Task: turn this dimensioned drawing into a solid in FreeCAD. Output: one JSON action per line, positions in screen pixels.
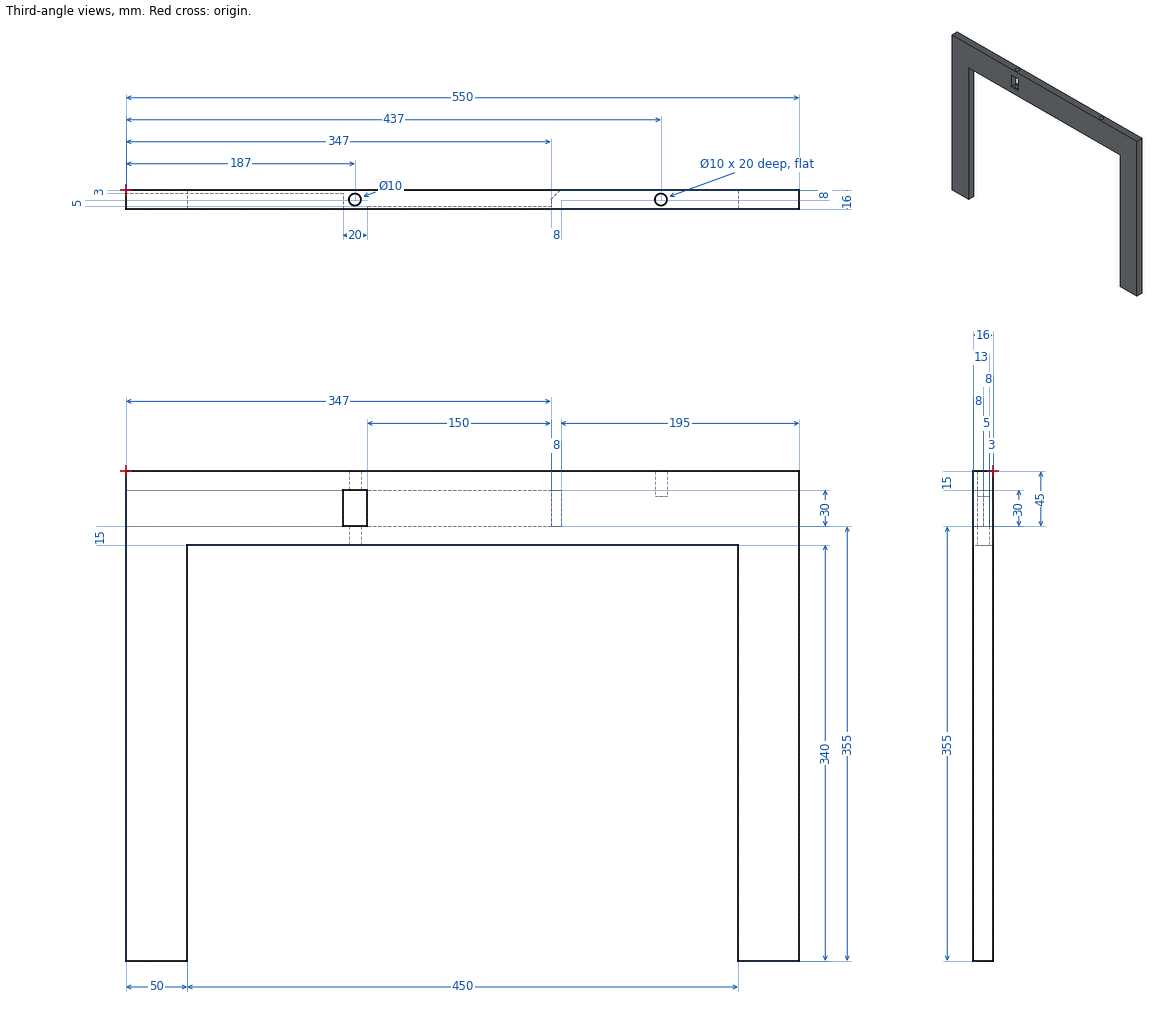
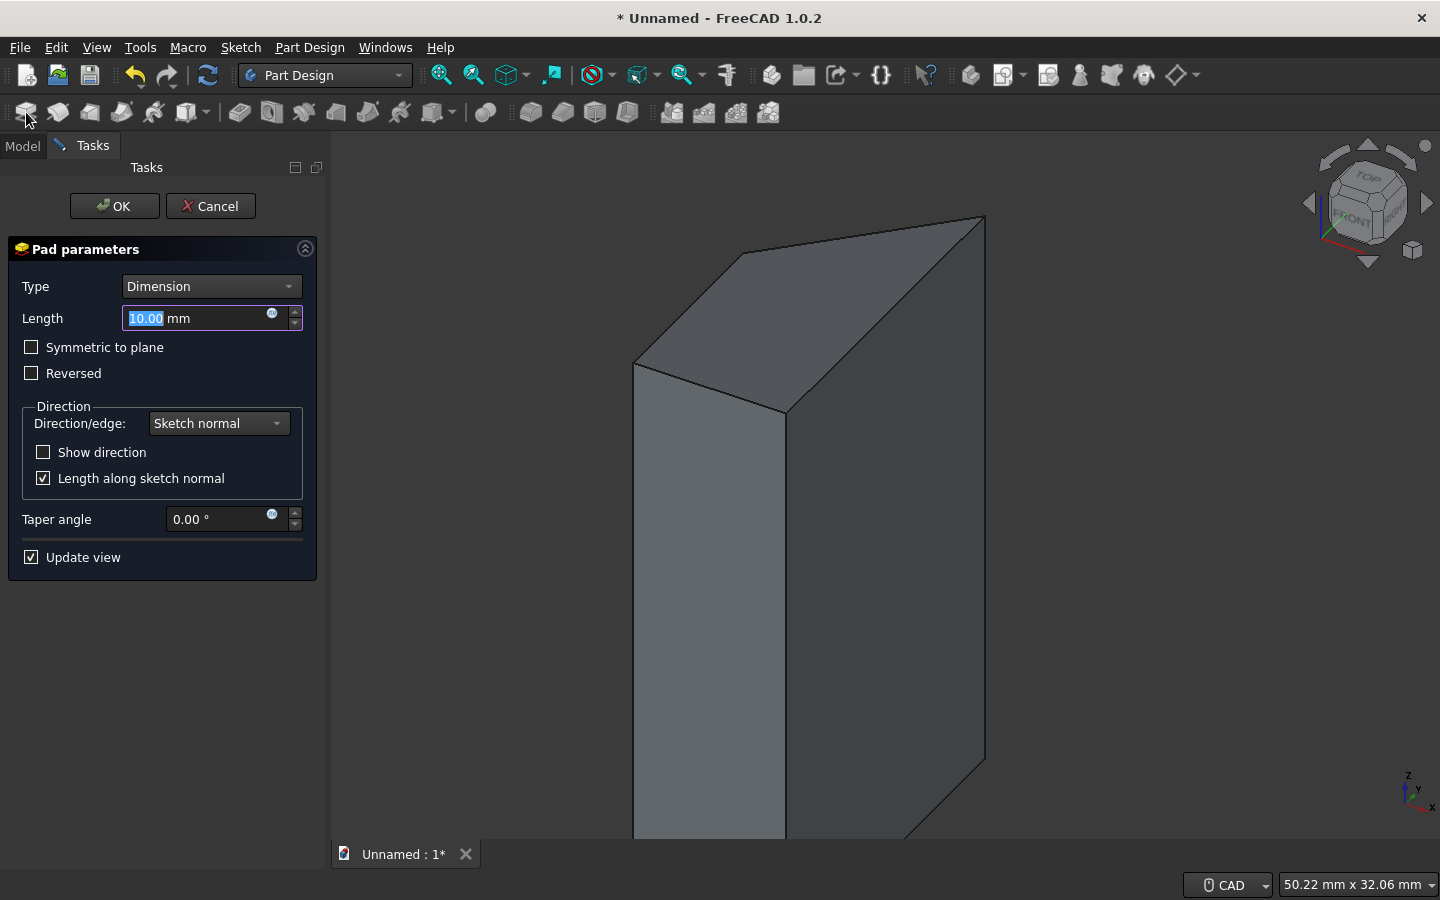
{"action": "type", "text": "8"}
{"action": "key", "text": "Tab"}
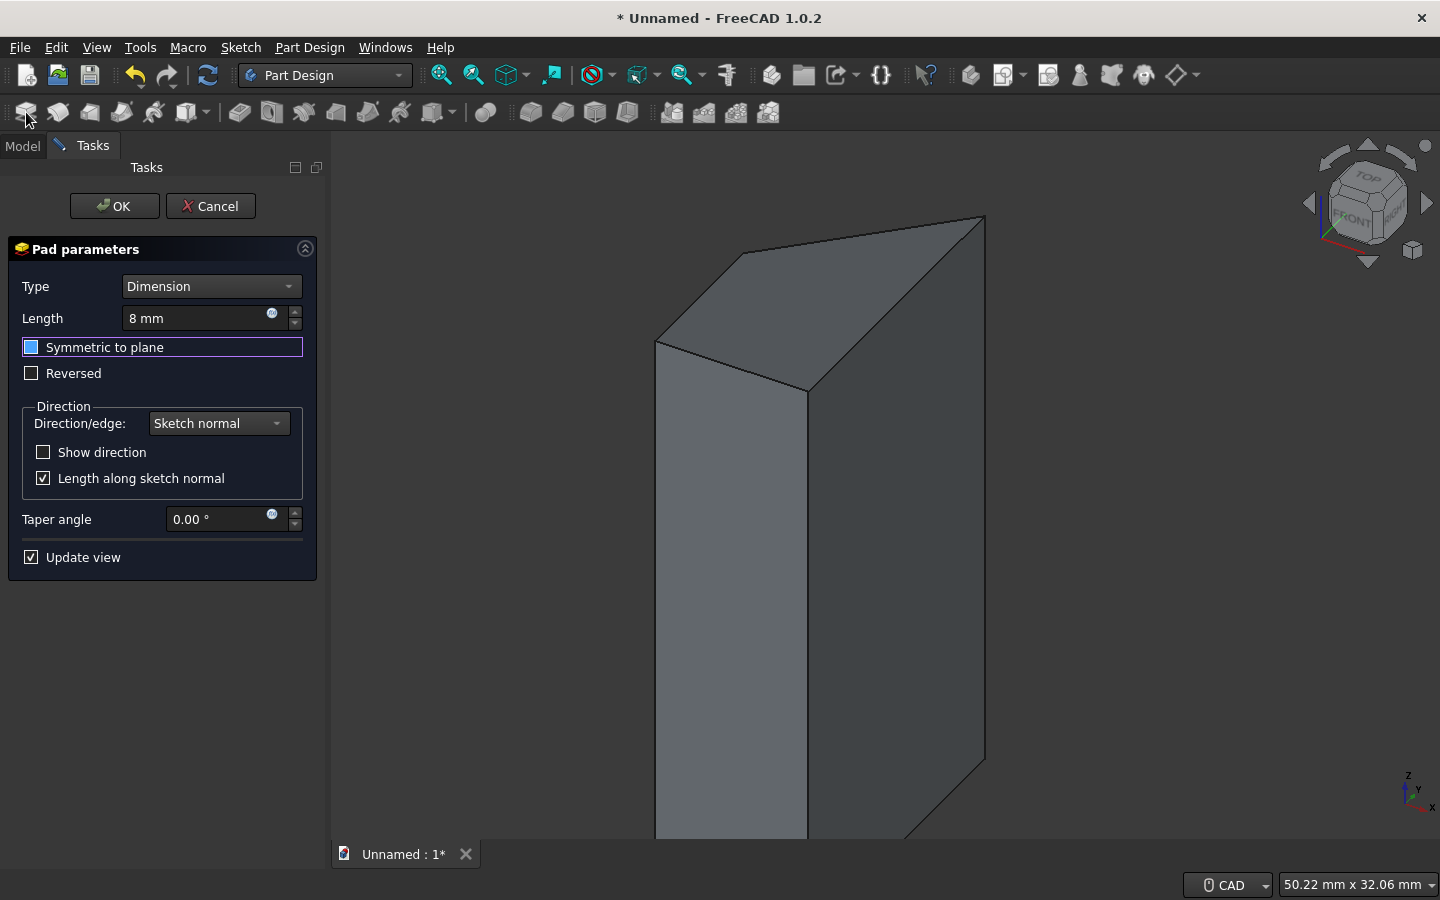
{"action": "left_click", "coordinate": [115, 206]}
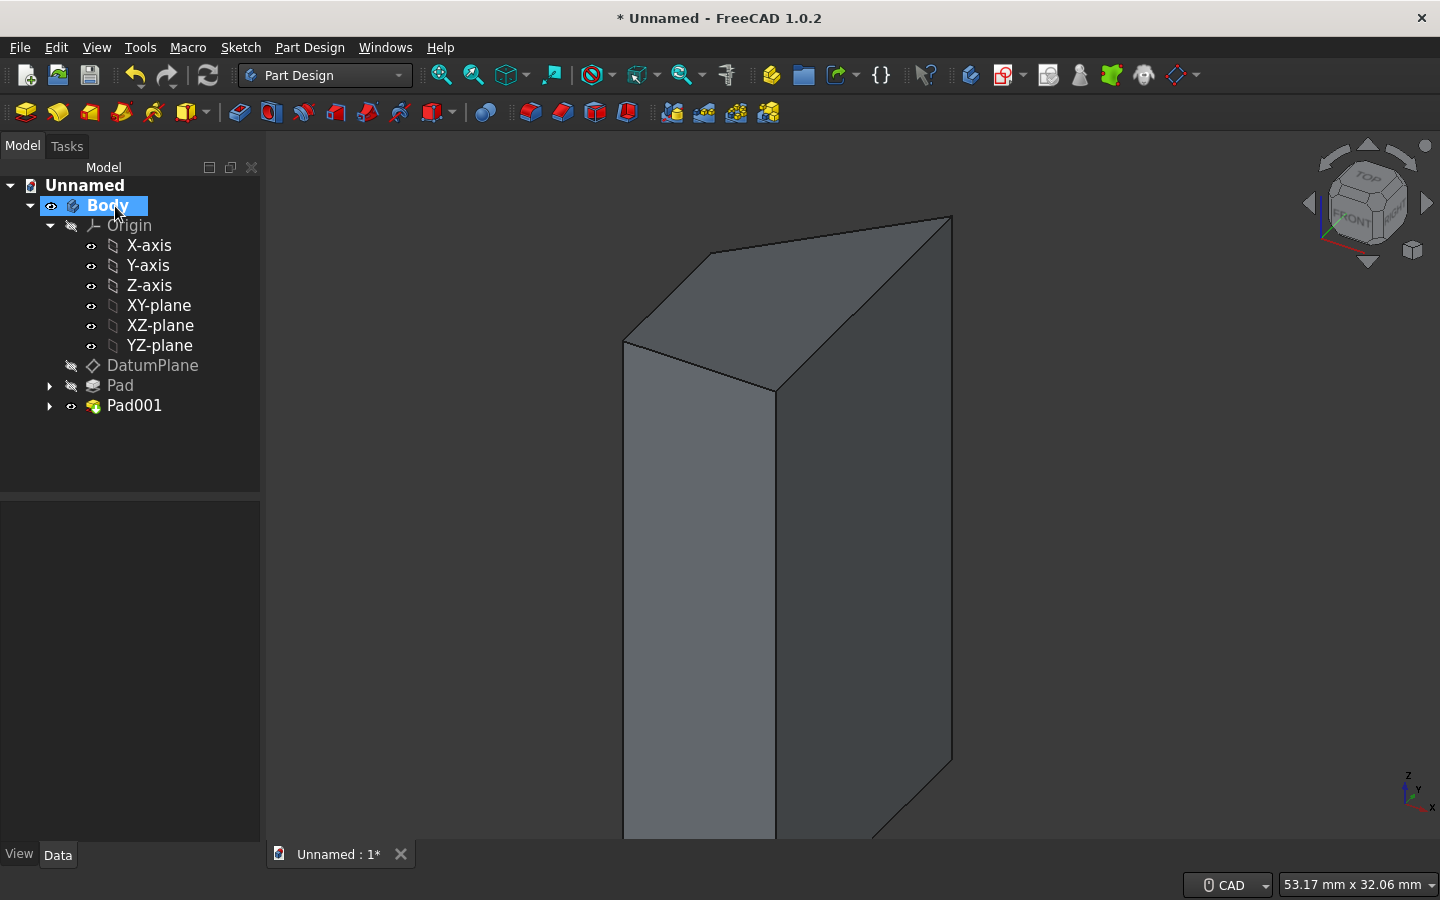
{"action": "left_click", "coordinate": [442, 76]}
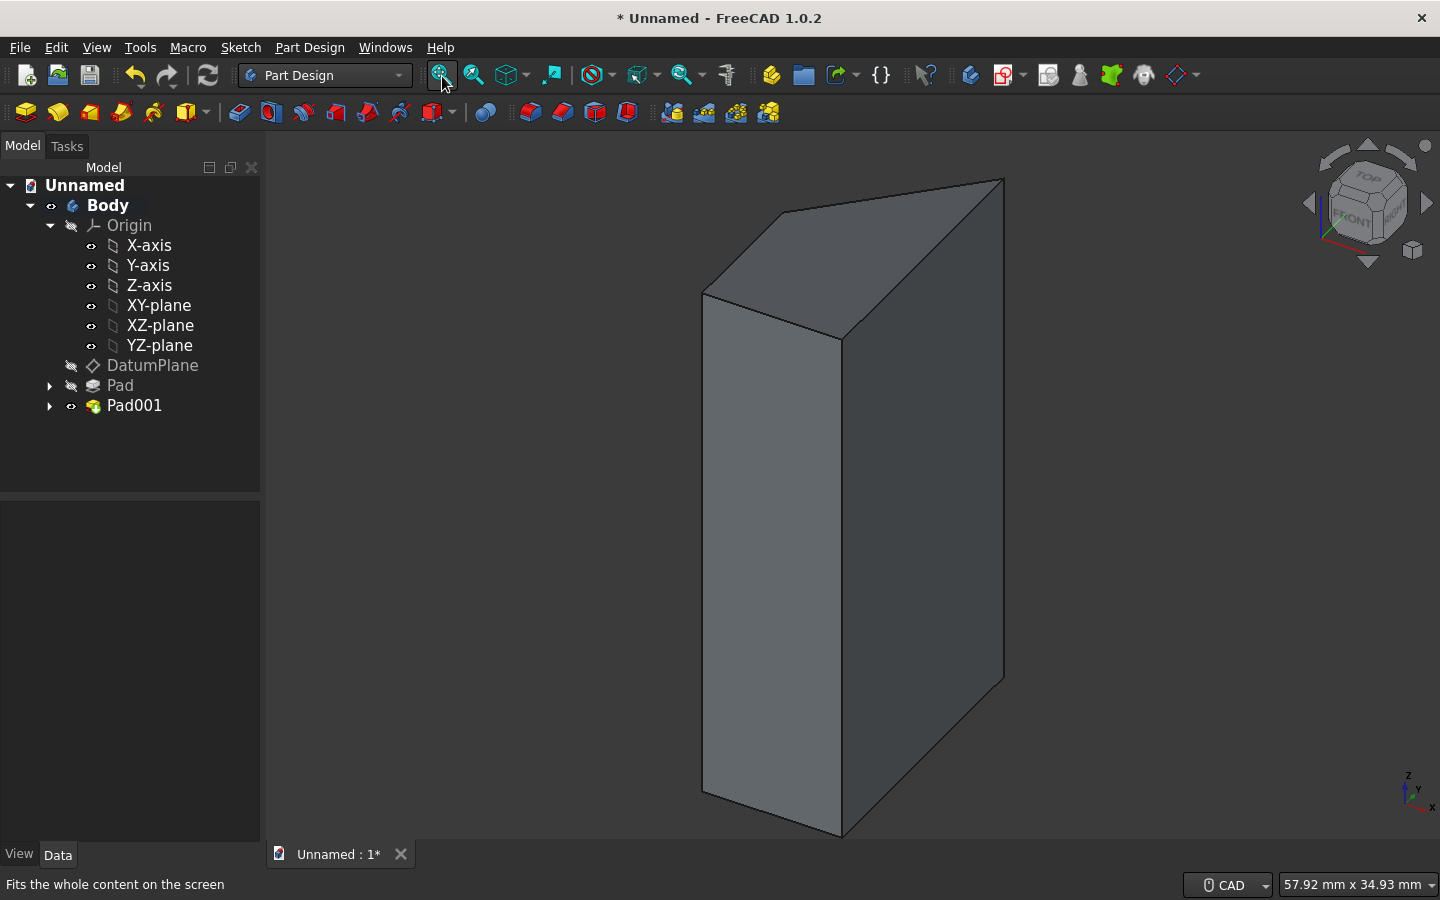
{"action": "left_click", "coordinate": [830, 258]}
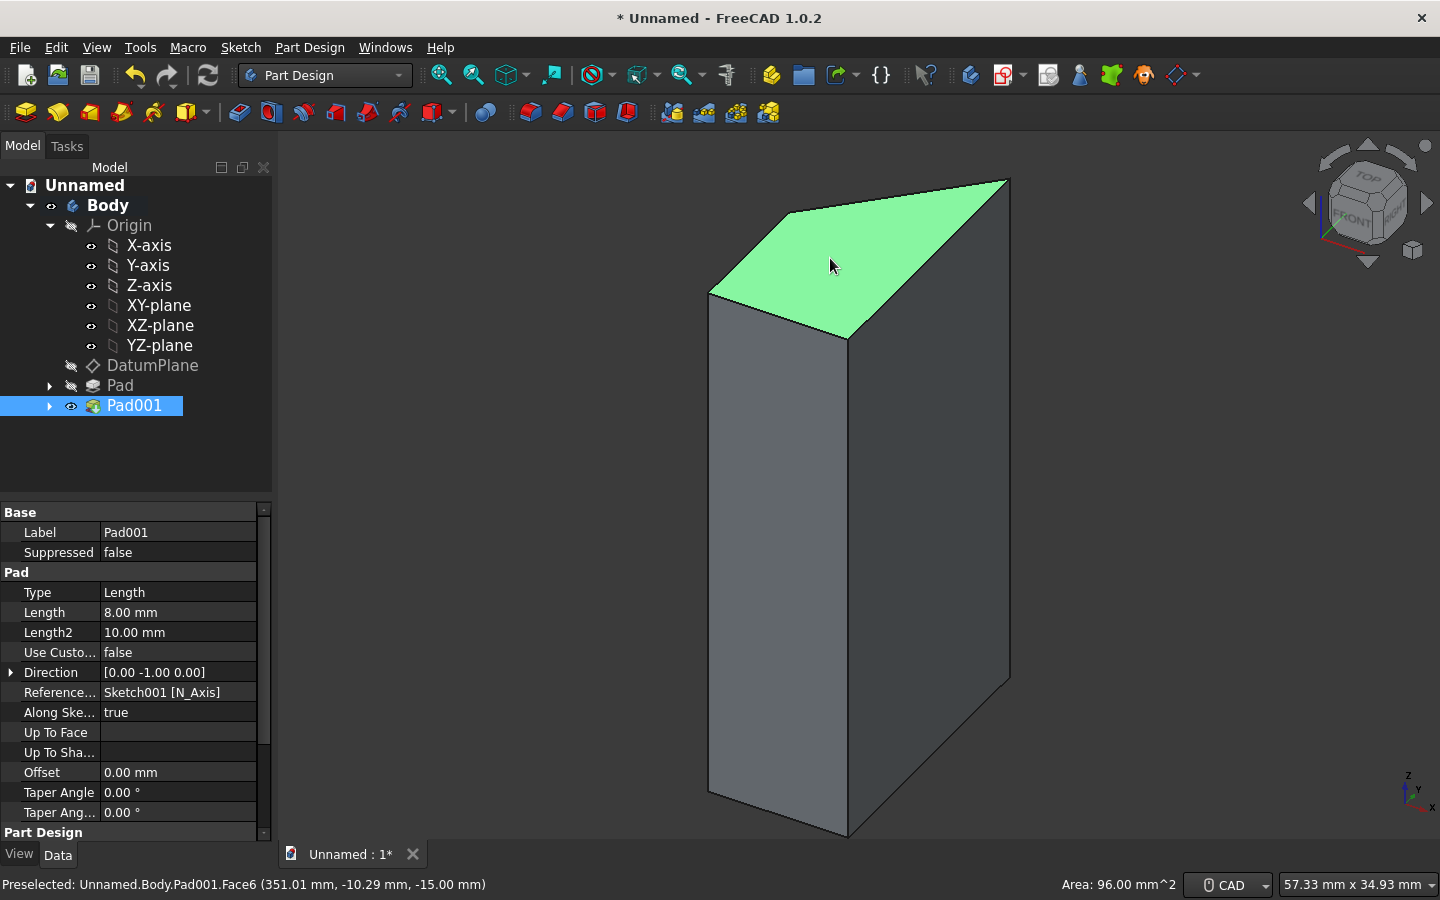
{"action": "left_click", "coordinate": [1004, 76]}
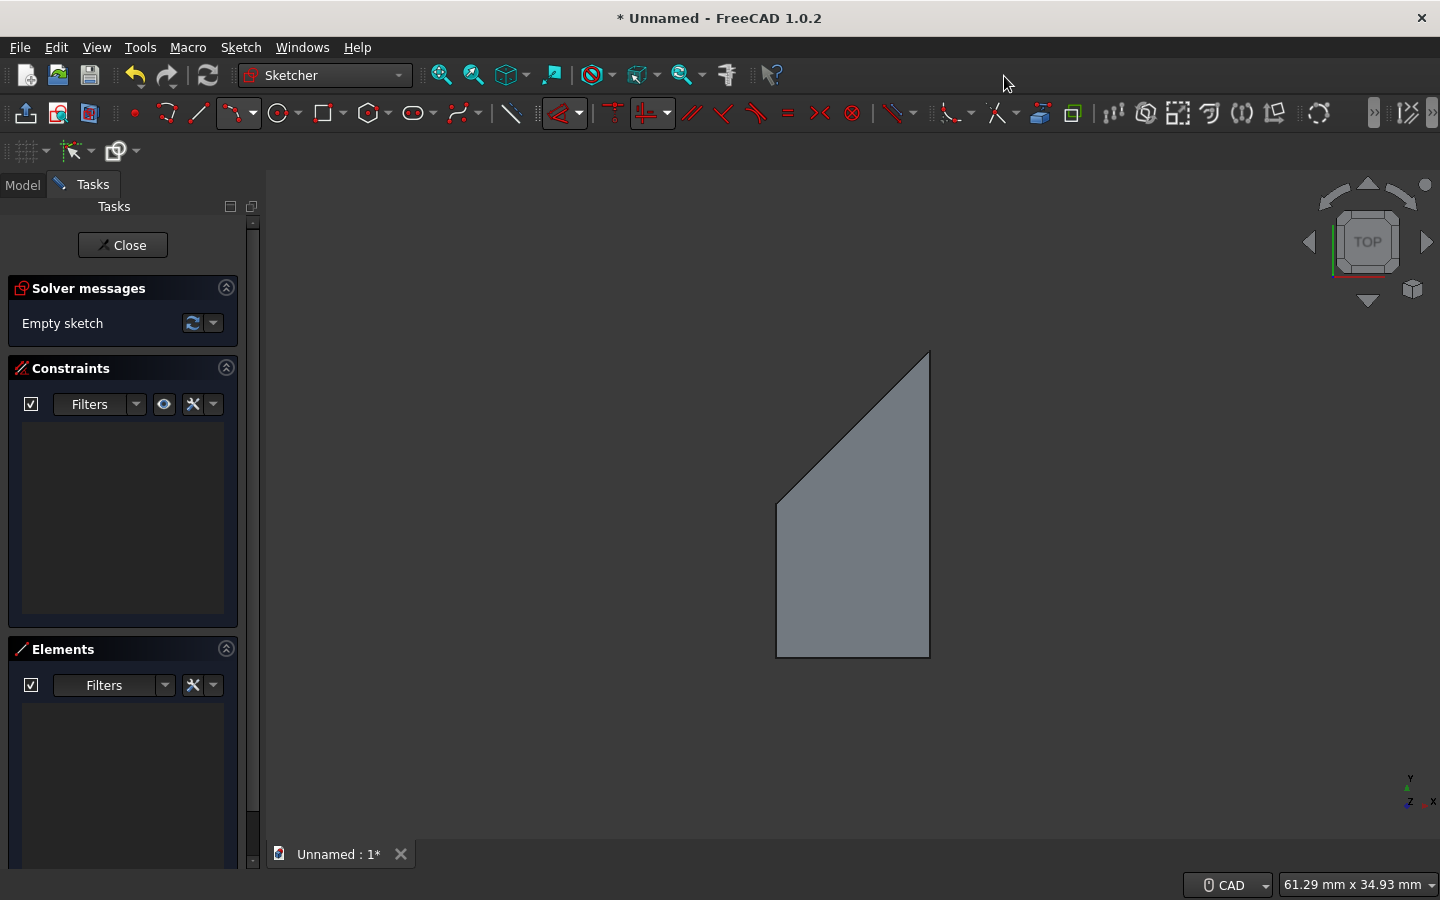
{"action": "scroll", "coordinate": [992, 504], "scroll_direction": "up", "scroll_amount": 2}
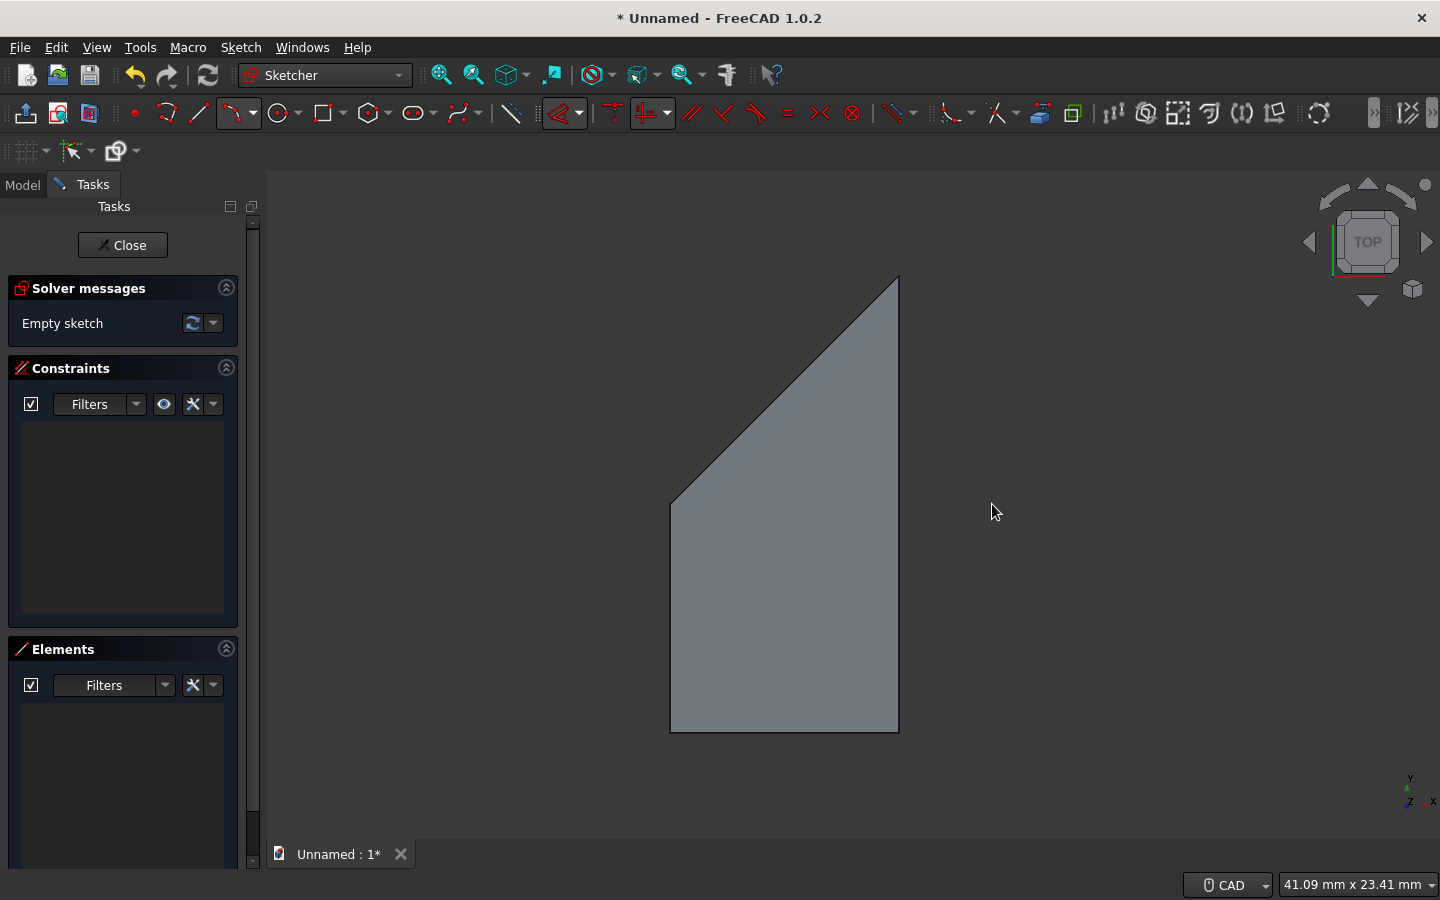
{"action": "left_click", "coordinate": [324, 114]}